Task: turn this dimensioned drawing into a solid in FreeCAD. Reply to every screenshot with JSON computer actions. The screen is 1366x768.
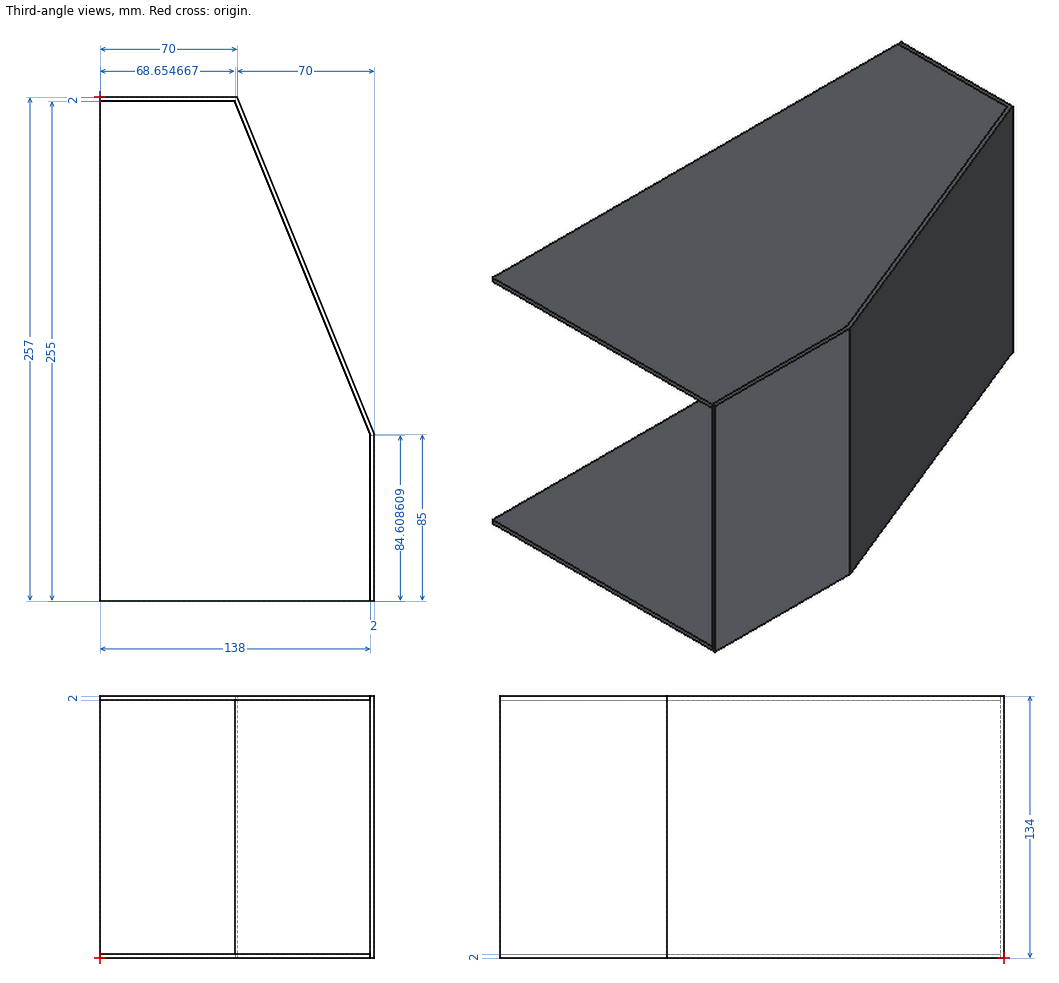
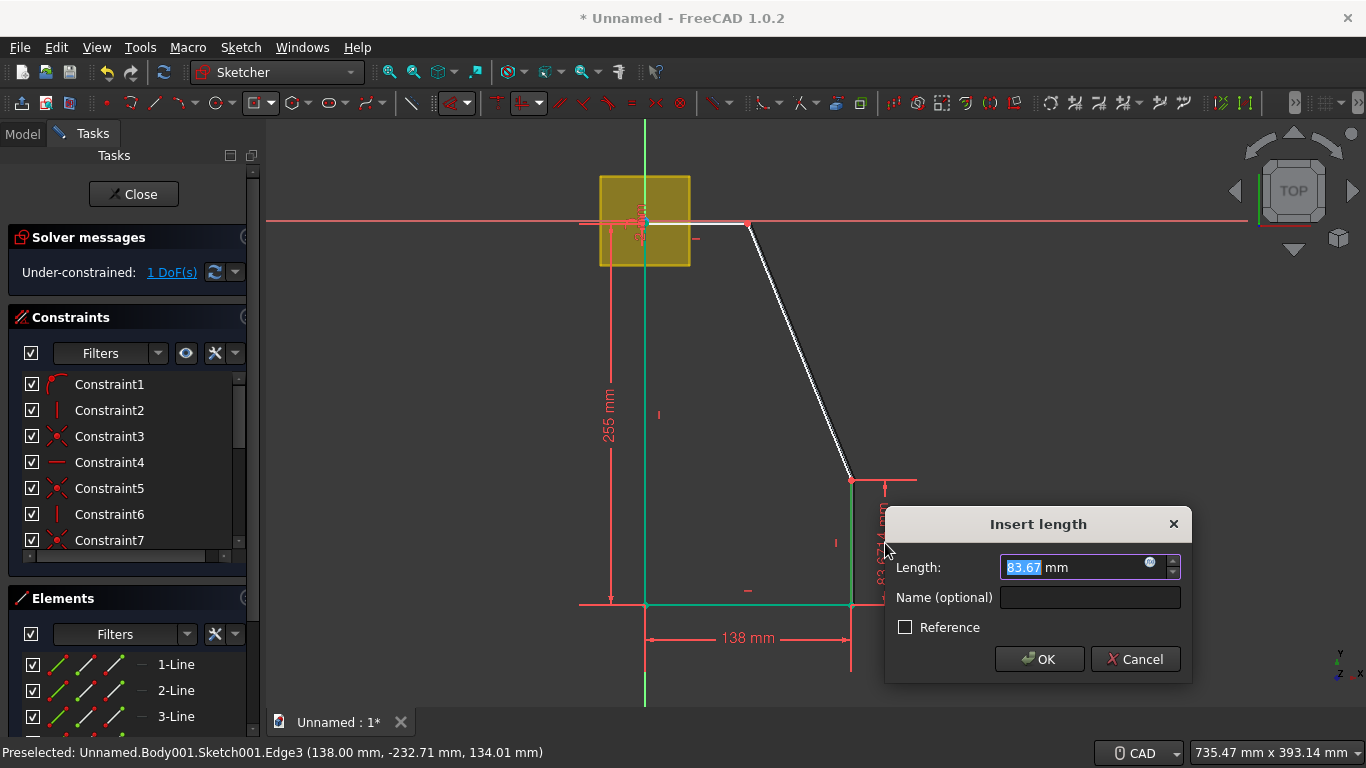
{"action": "type", "text": "84.608609"}
{"action": "key", "text": "Return"}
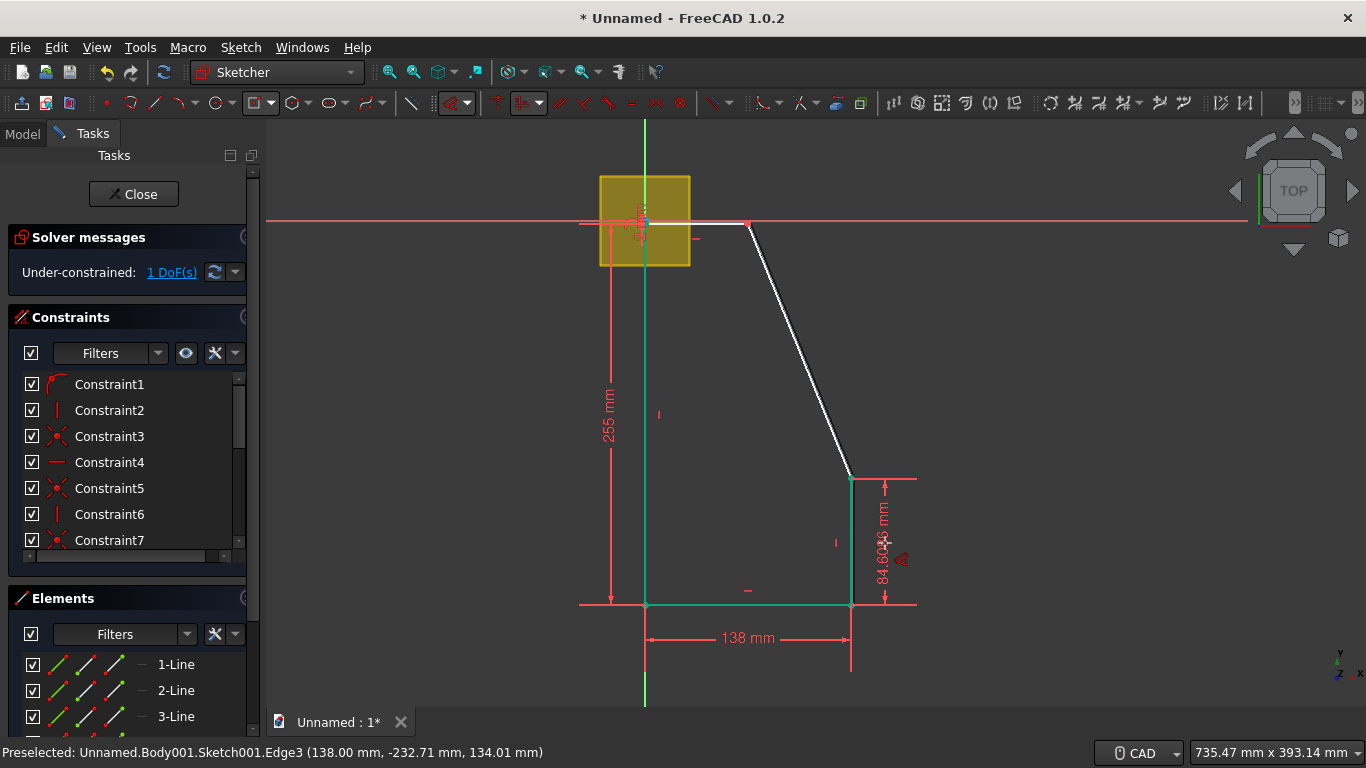
{"action": "left_click", "coordinate": [717, 224]}
{"action": "left_click", "coordinate": [696, 190]}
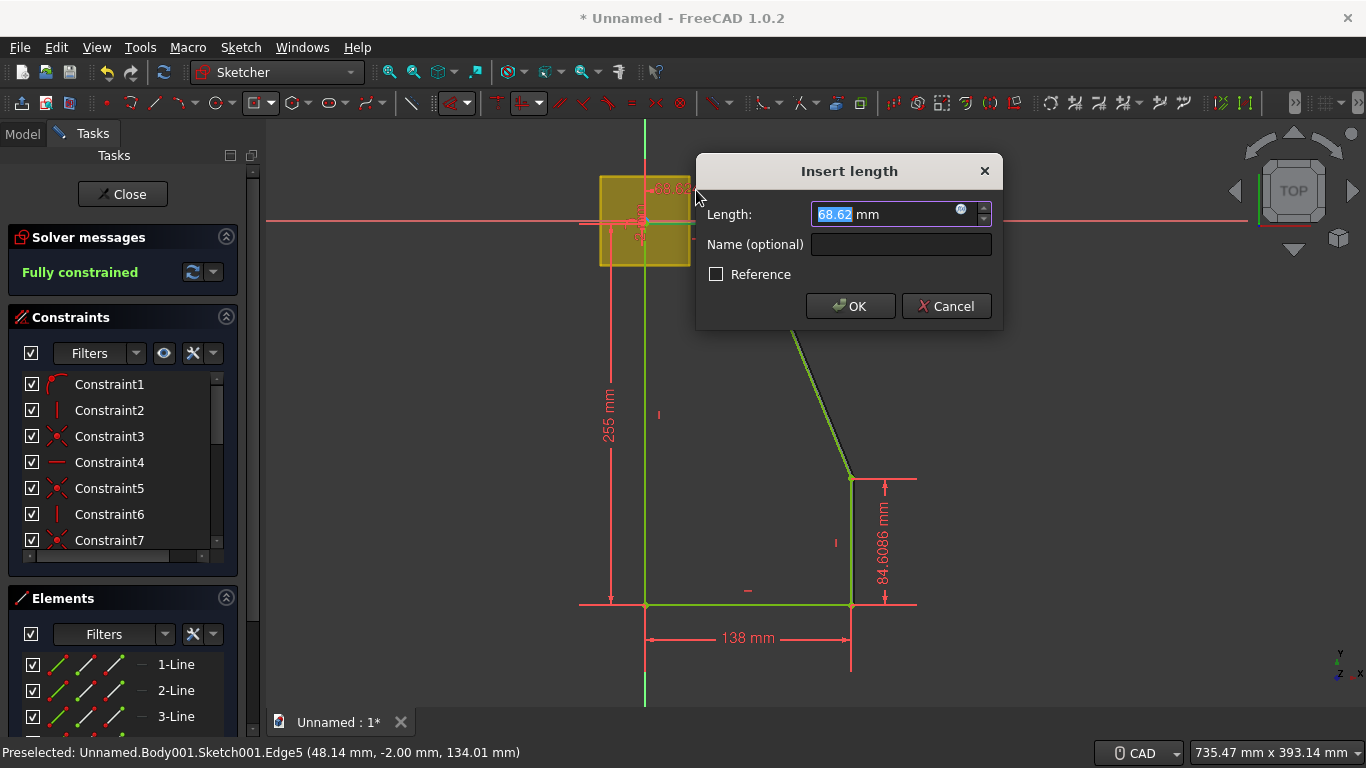
{"action": "type", "text": "68.654667"}
{"action": "key", "text": "Return"}
{"action": "key", "text": "Escape"}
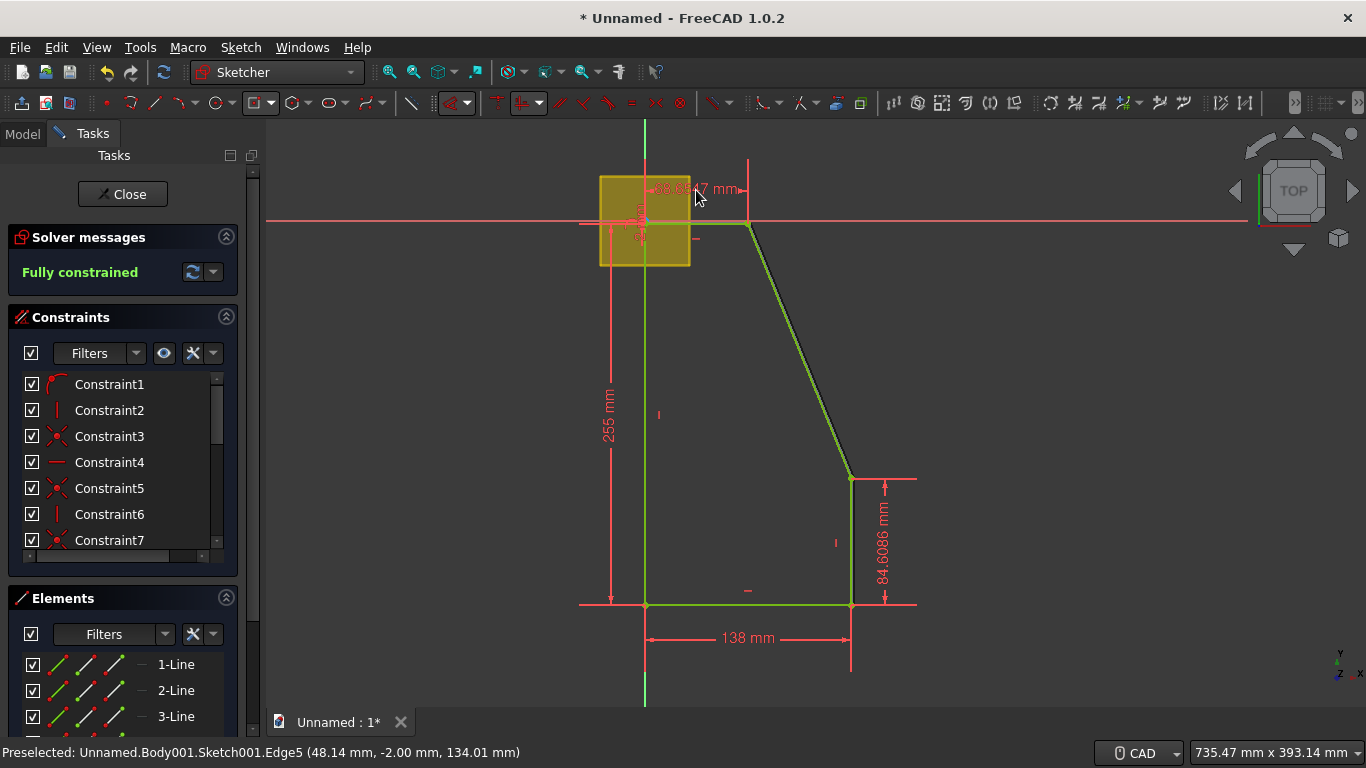
{"action": "left_click", "coordinate": [123, 194]}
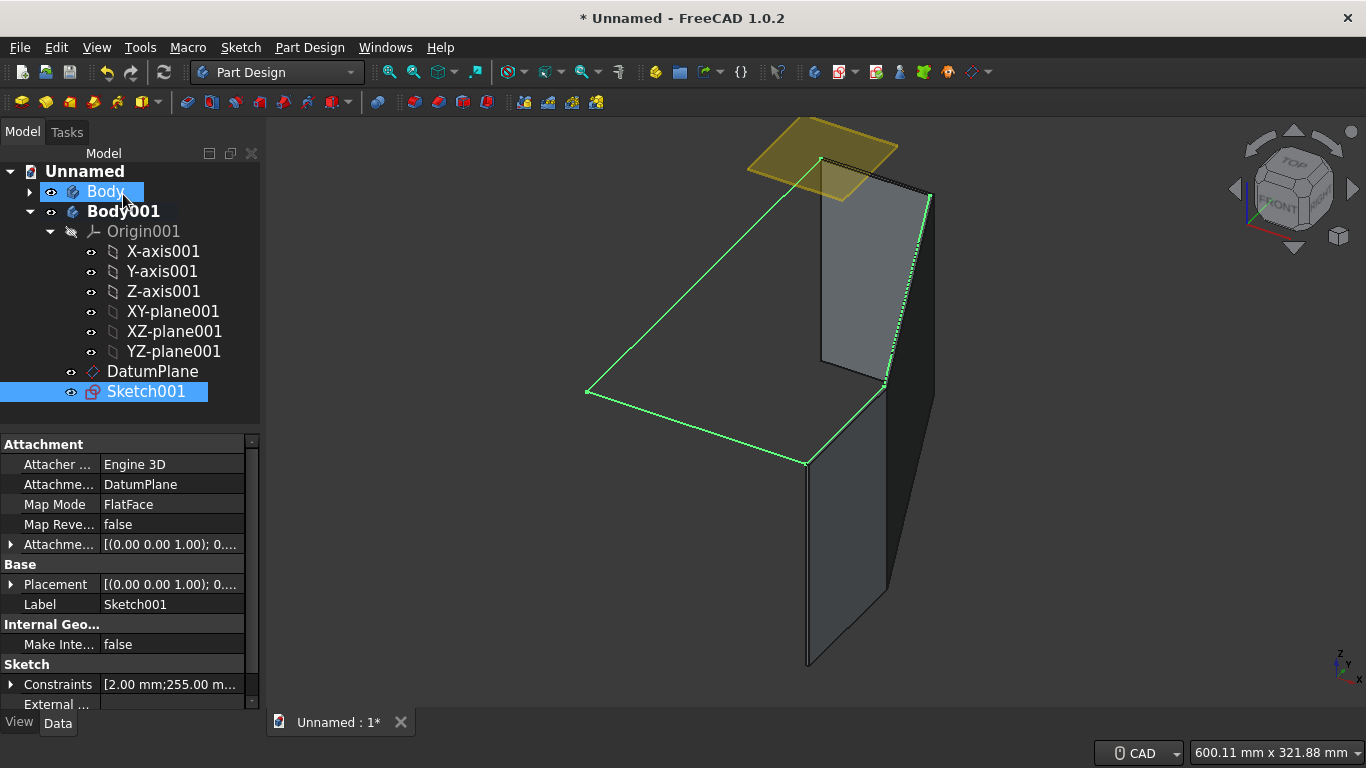
{"action": "left_click", "coordinate": [22, 102]}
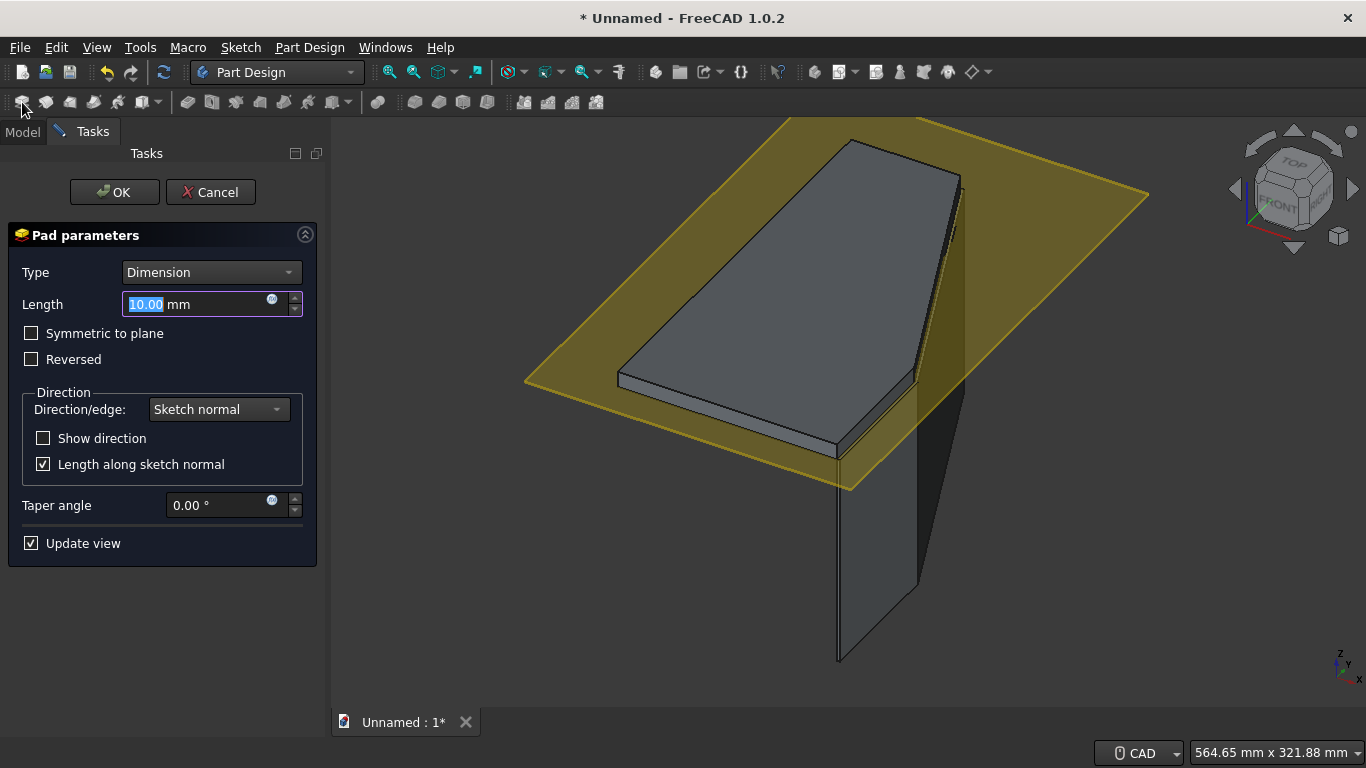
{"action": "type", "text": "2"}
{"action": "key", "text": "Tab"}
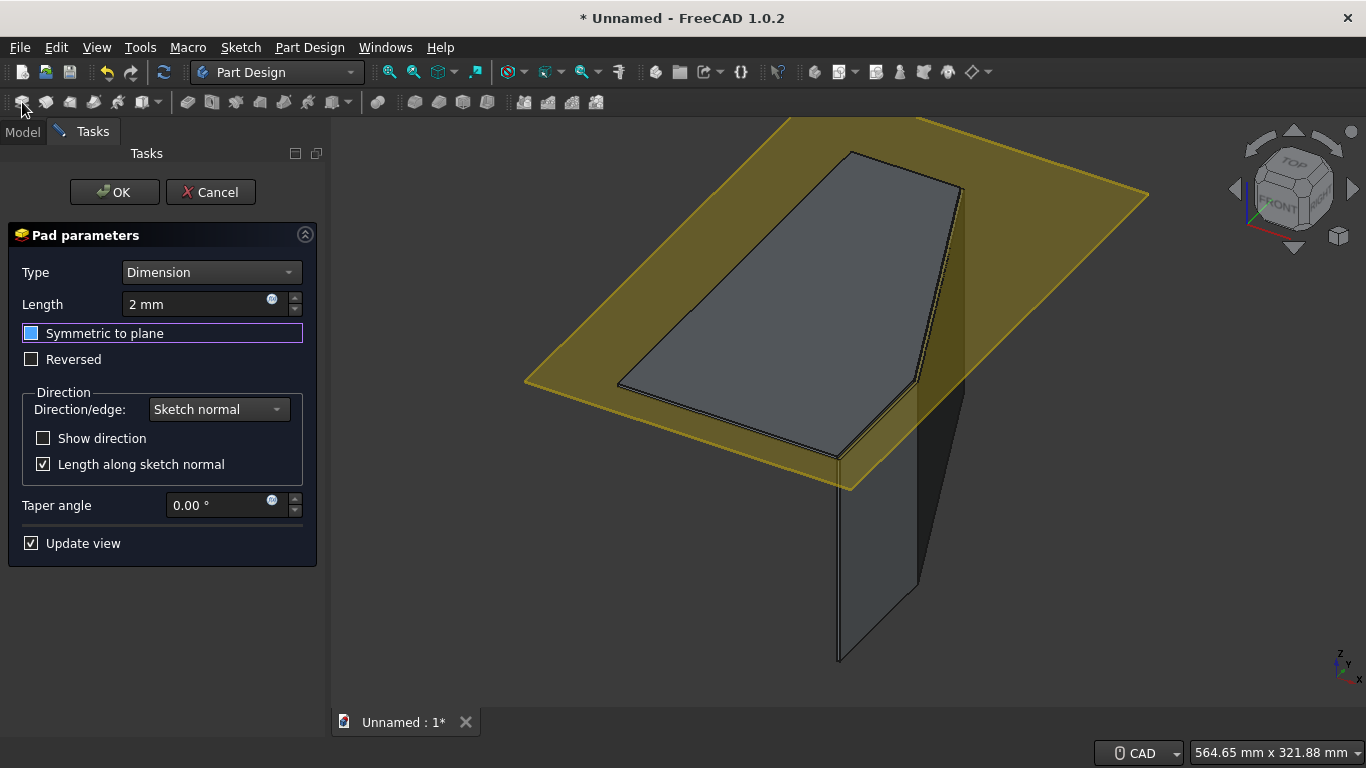
{"action": "left_click", "coordinate": [30, 359]}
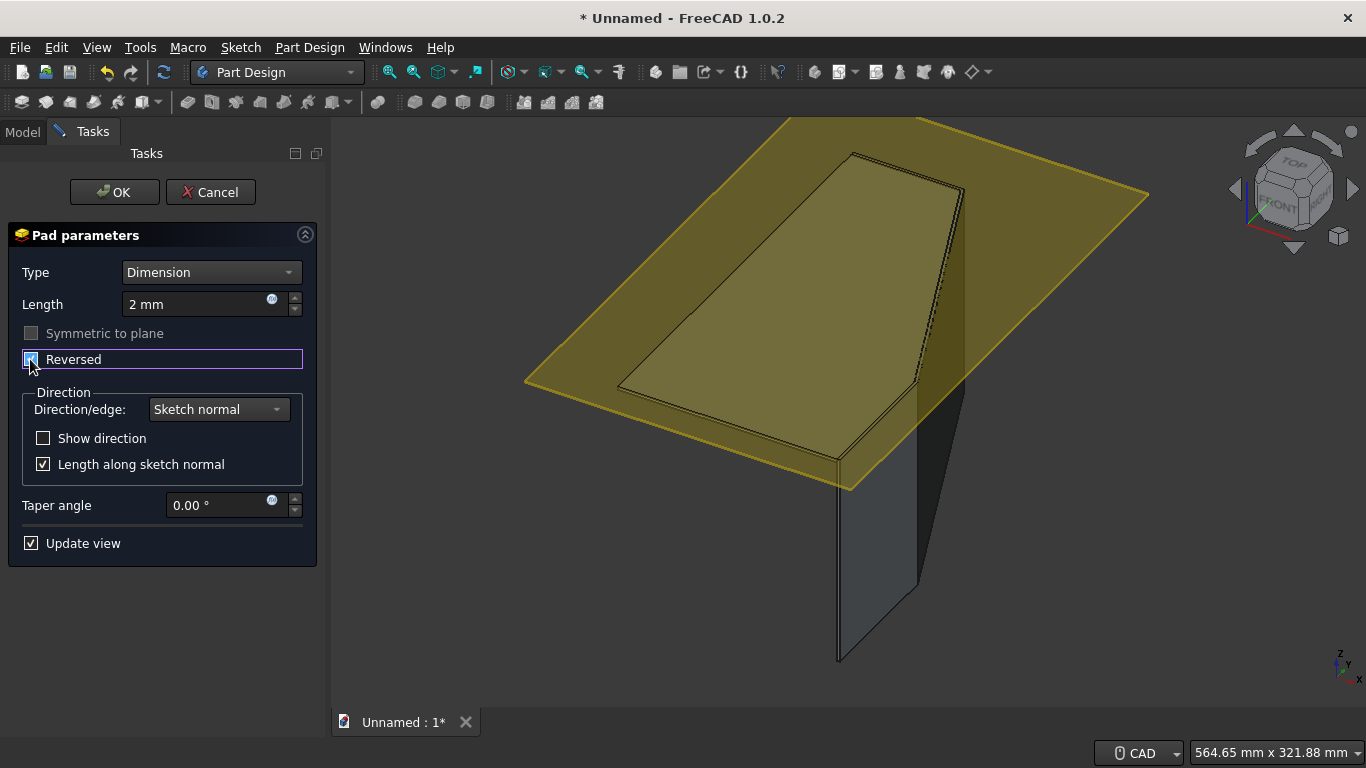
{"action": "left_click", "coordinate": [115, 192]}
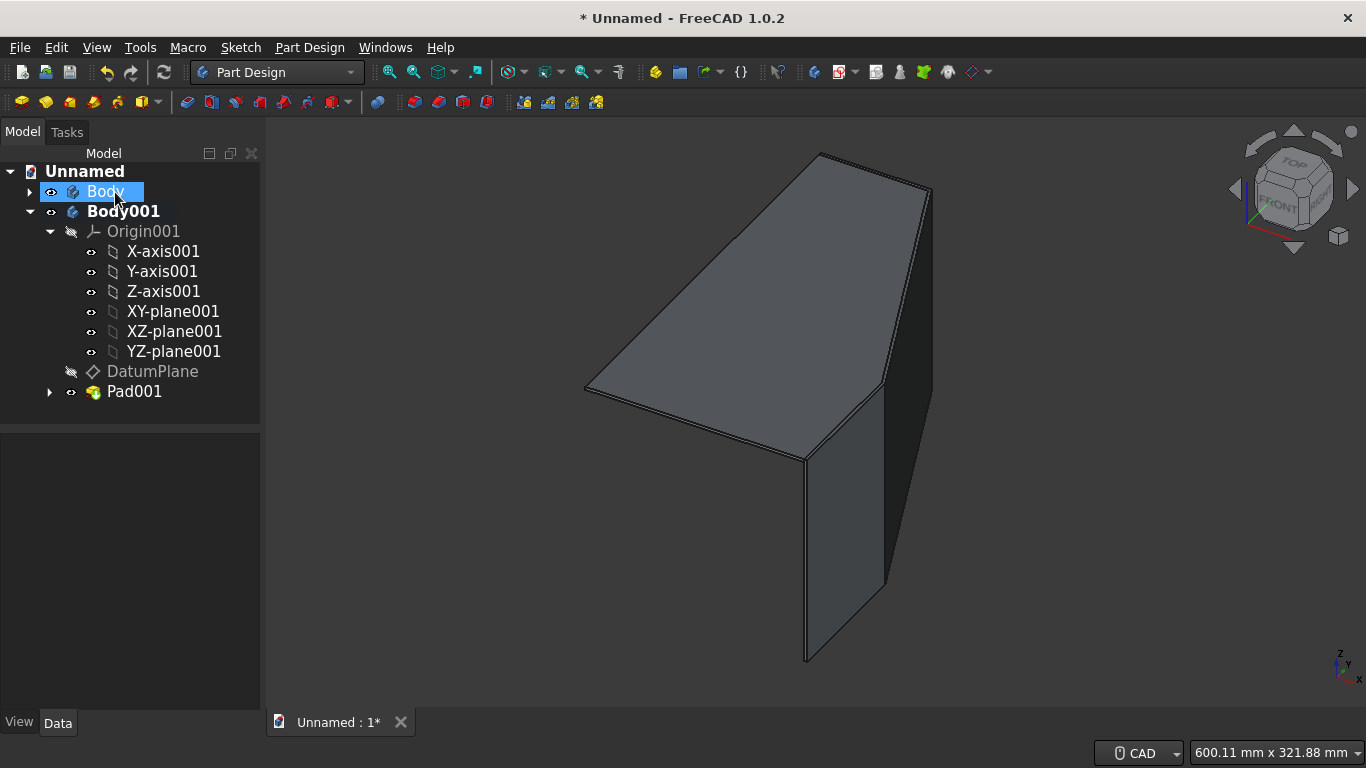
{"action": "left_click", "coordinate": [816, 72]}